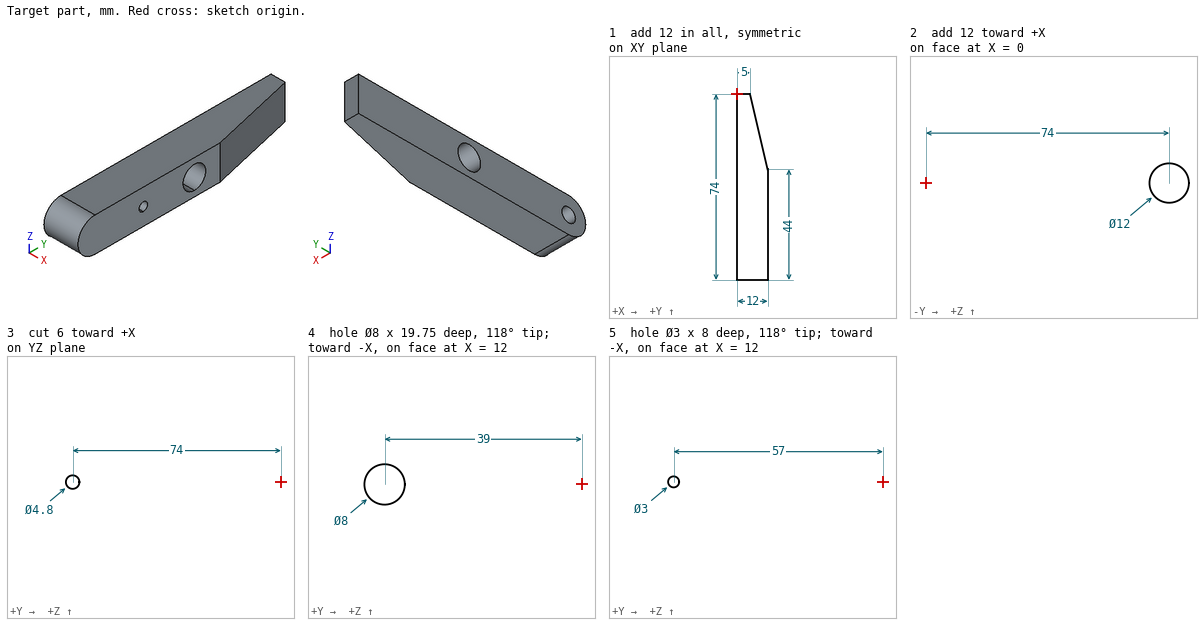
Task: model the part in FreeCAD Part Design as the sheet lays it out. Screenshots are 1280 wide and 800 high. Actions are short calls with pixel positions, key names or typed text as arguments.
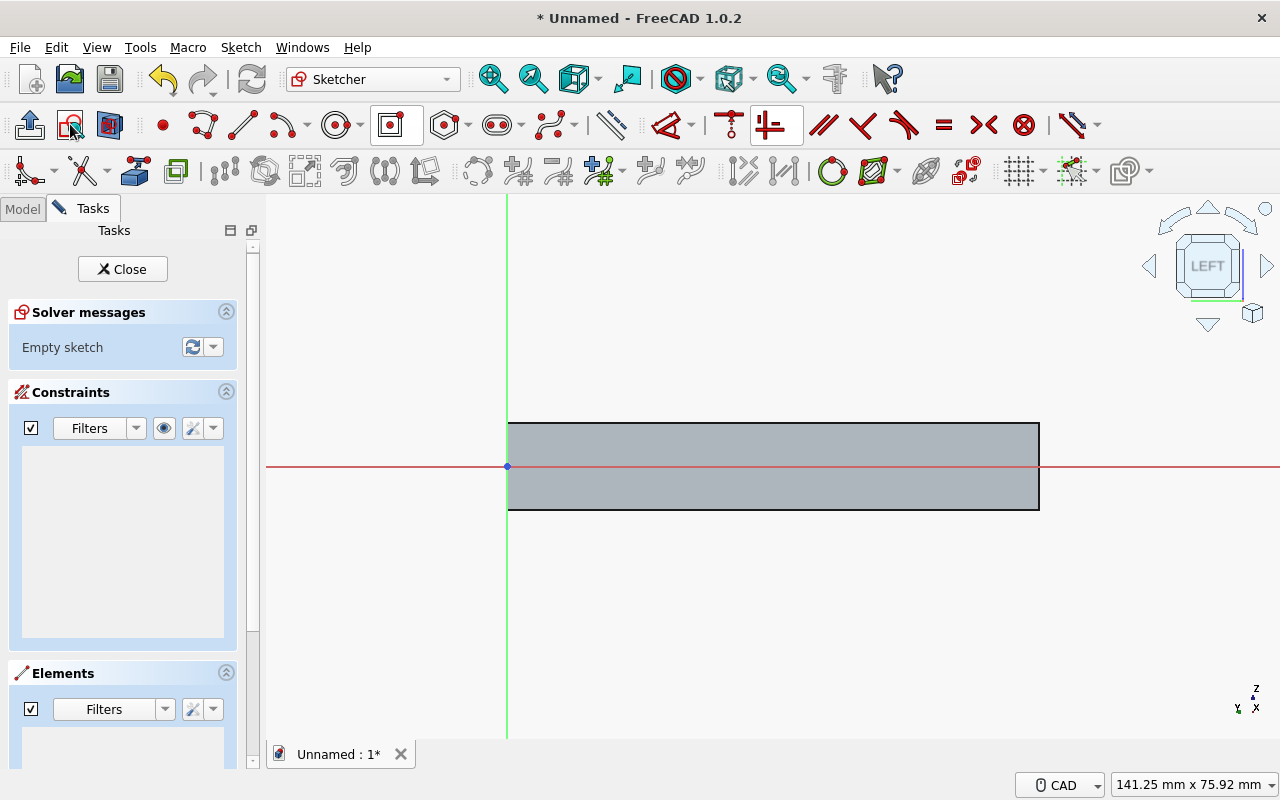
scroll(1115, 466, up, 7)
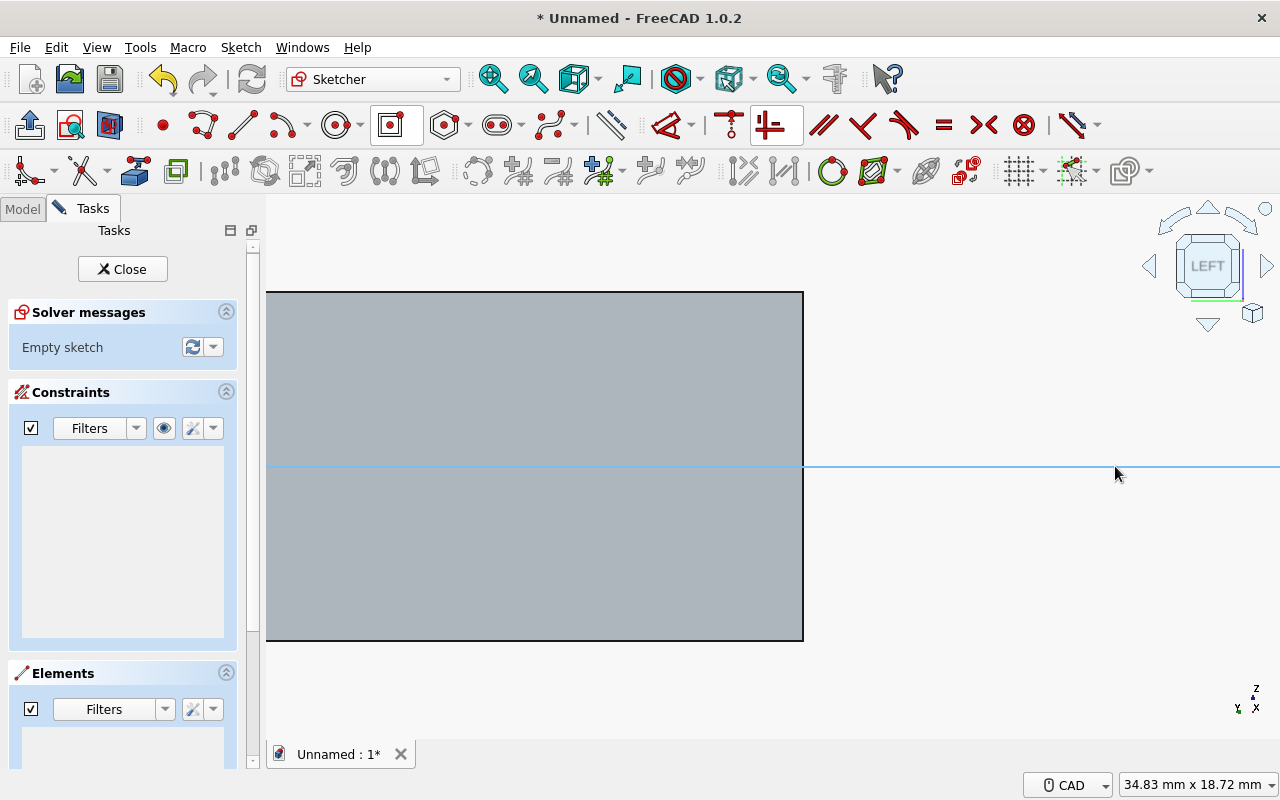
click(336, 126)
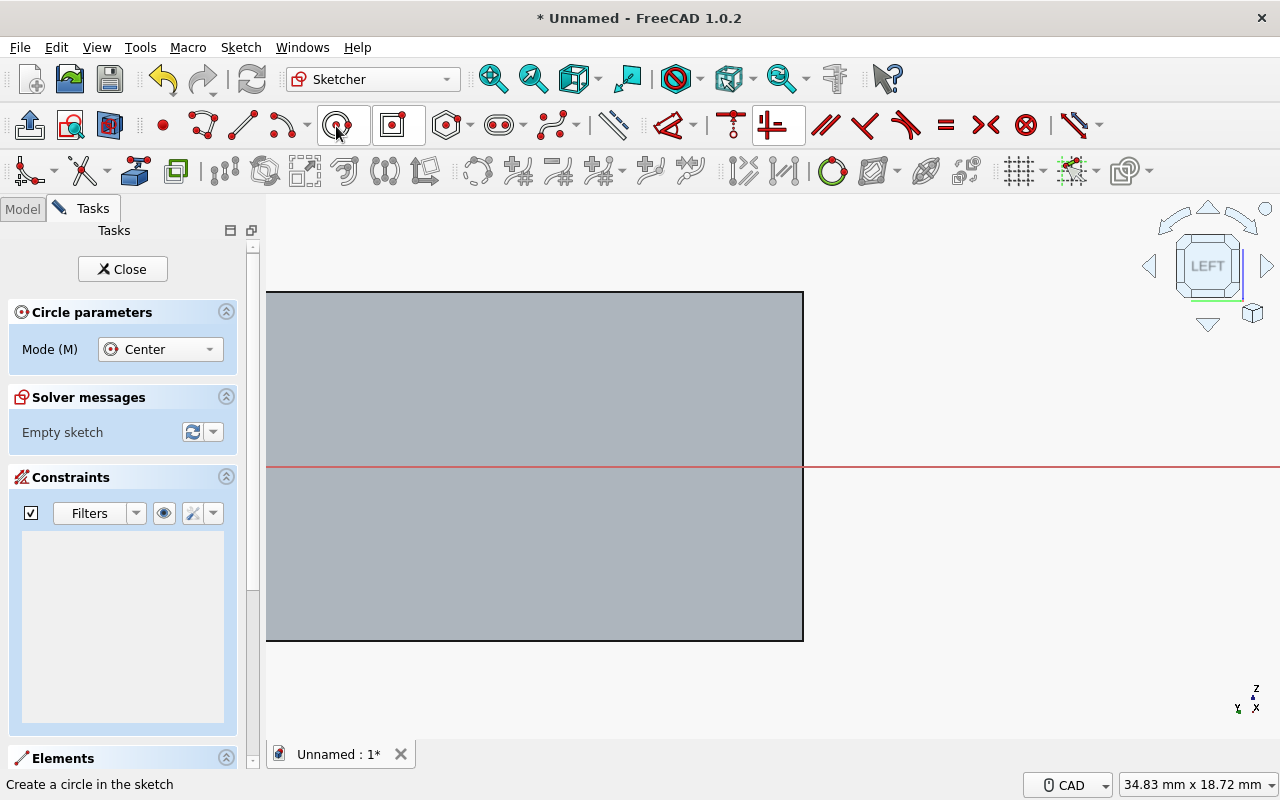
click(803, 466)
move(926, 343)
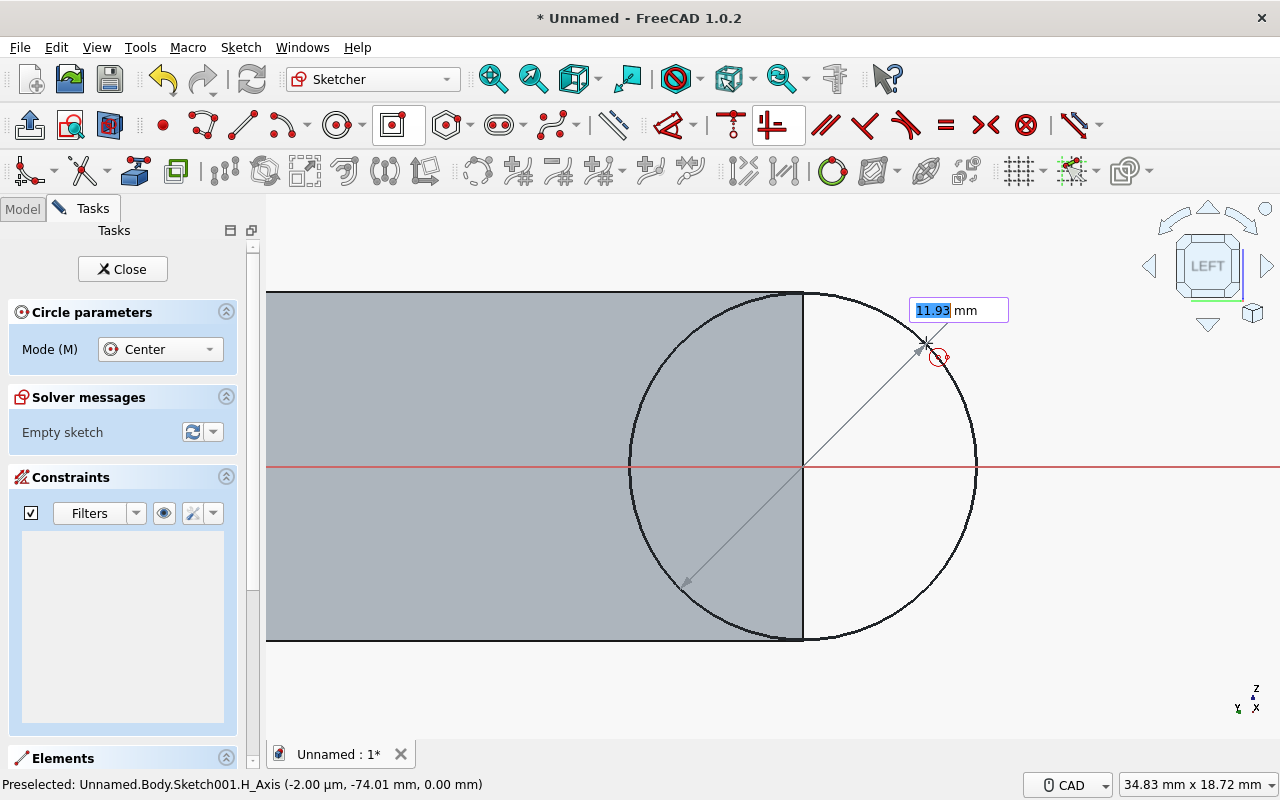
text(12)
key(Return)
key(Escape)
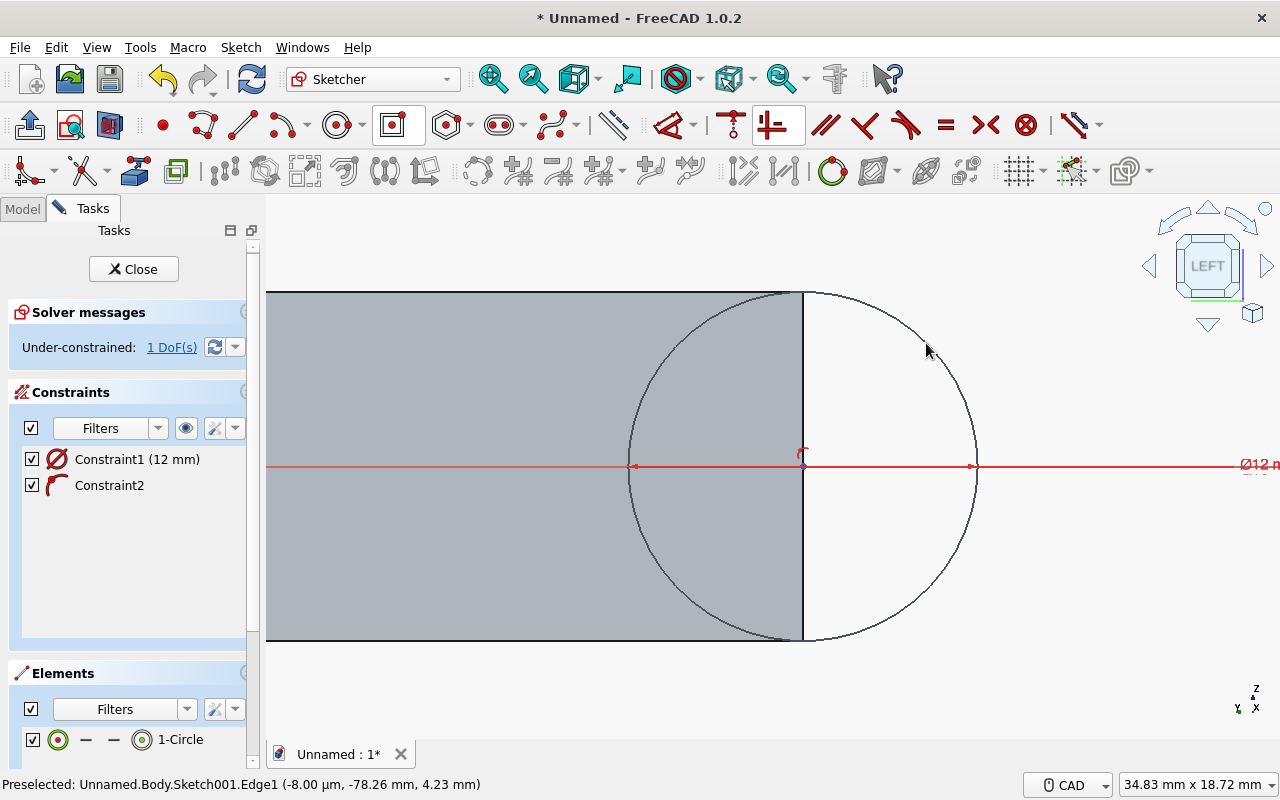
click(668, 126)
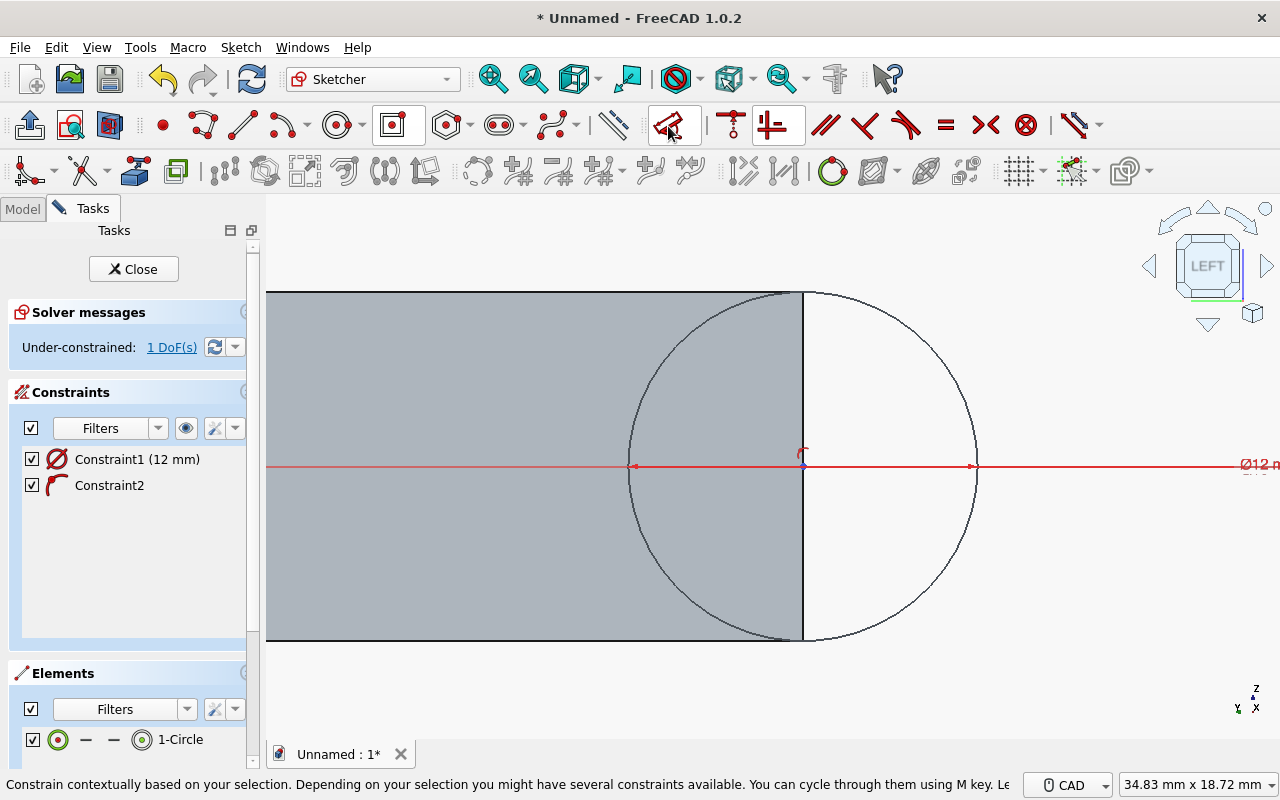
click(803, 466)
click(549, 500)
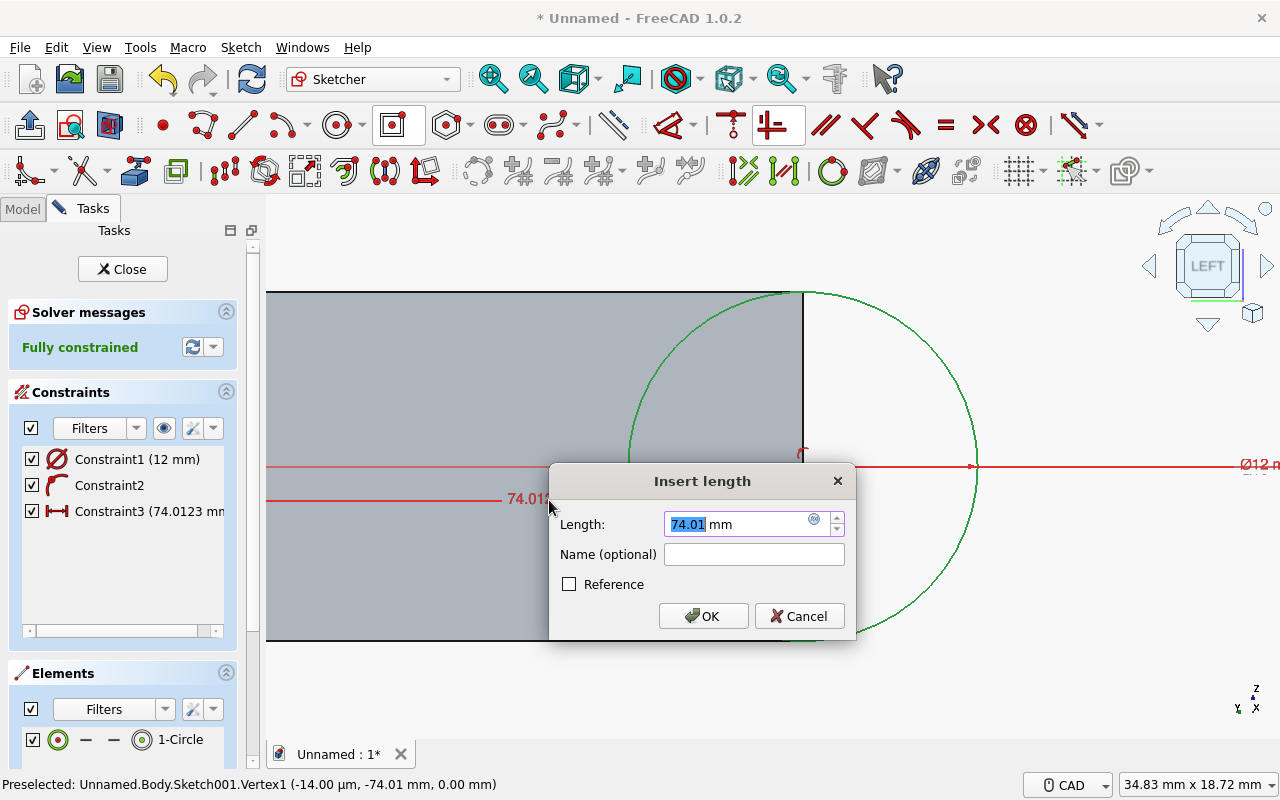
text(74)
key(Return)
key(Escape)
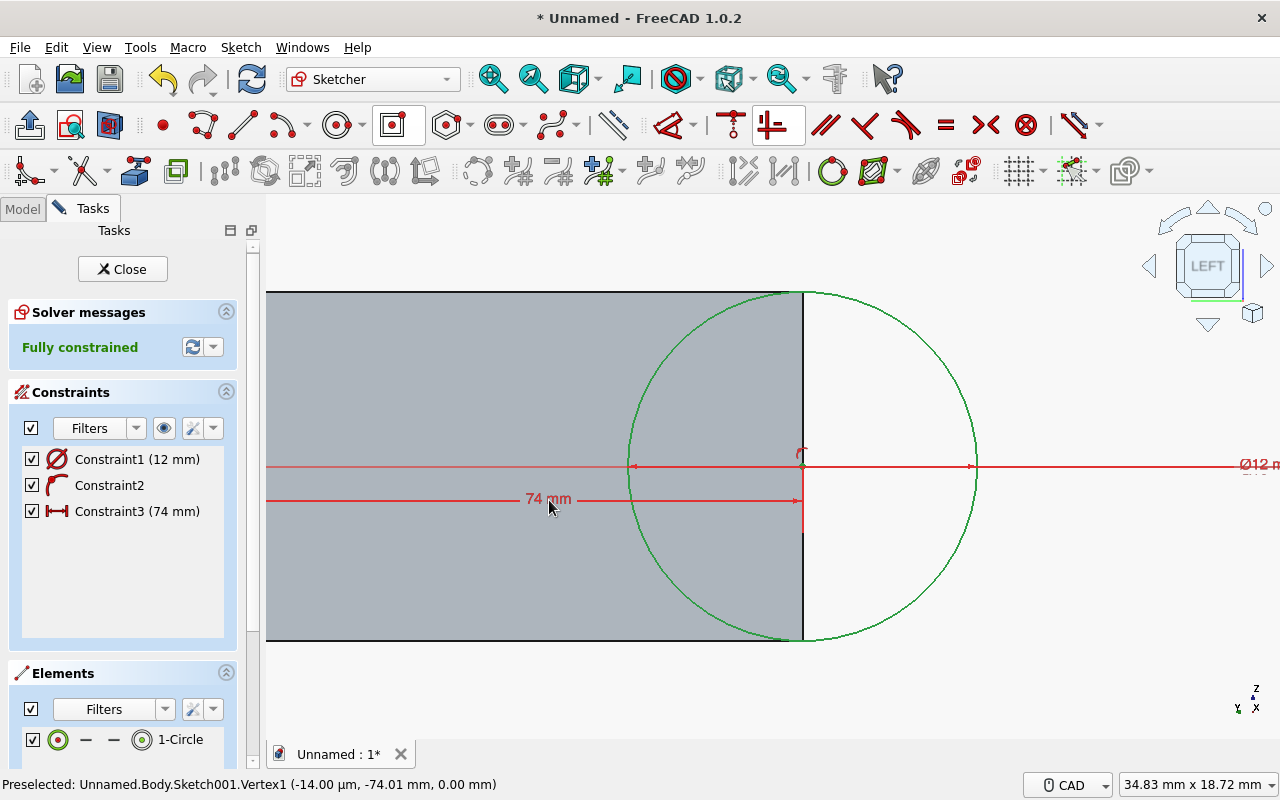
click(123, 269)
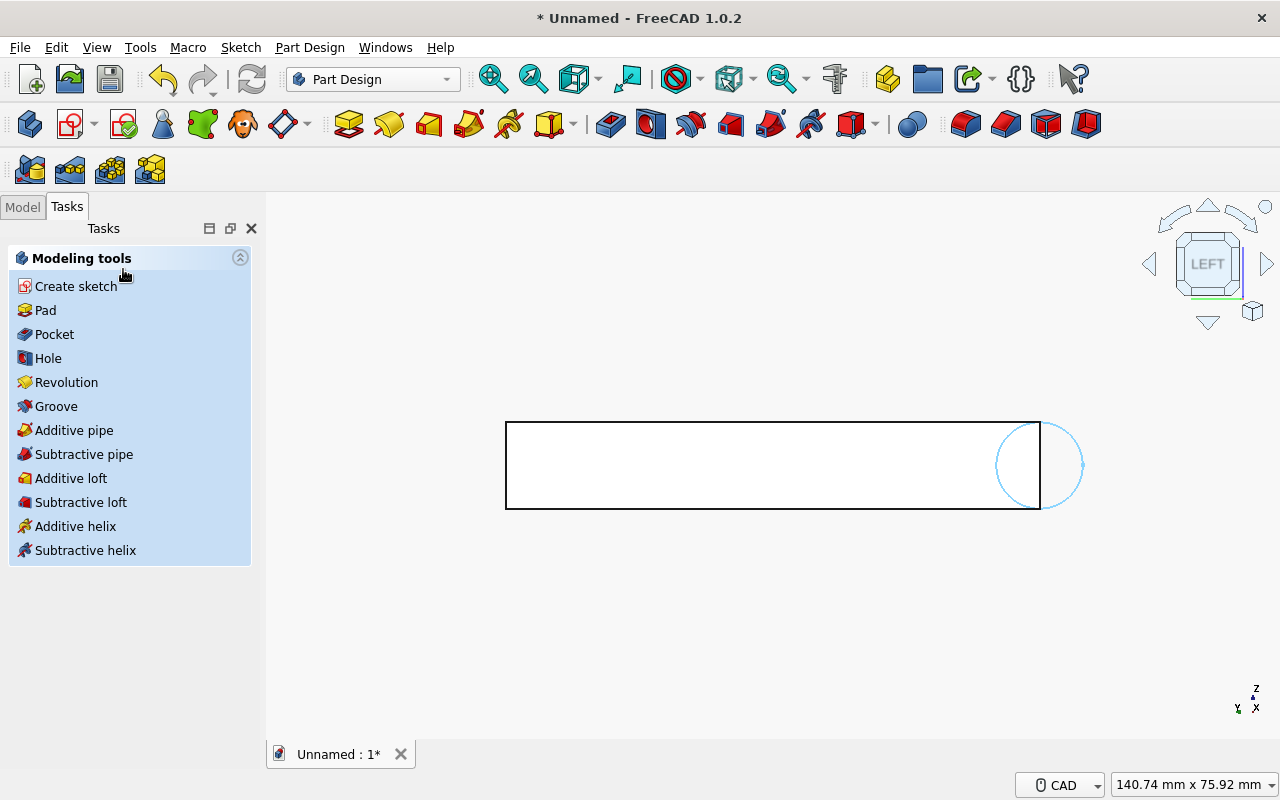
click(350, 124)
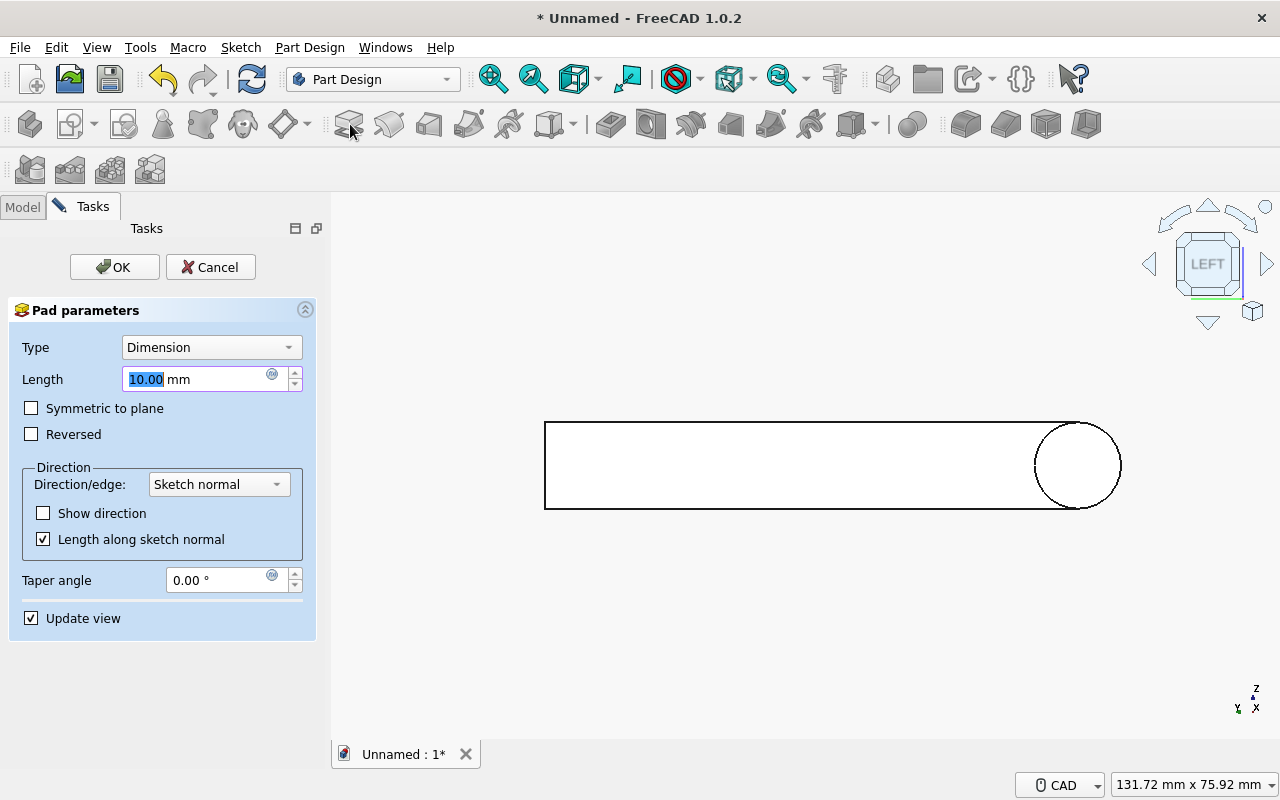
text(12)
key(Tab)